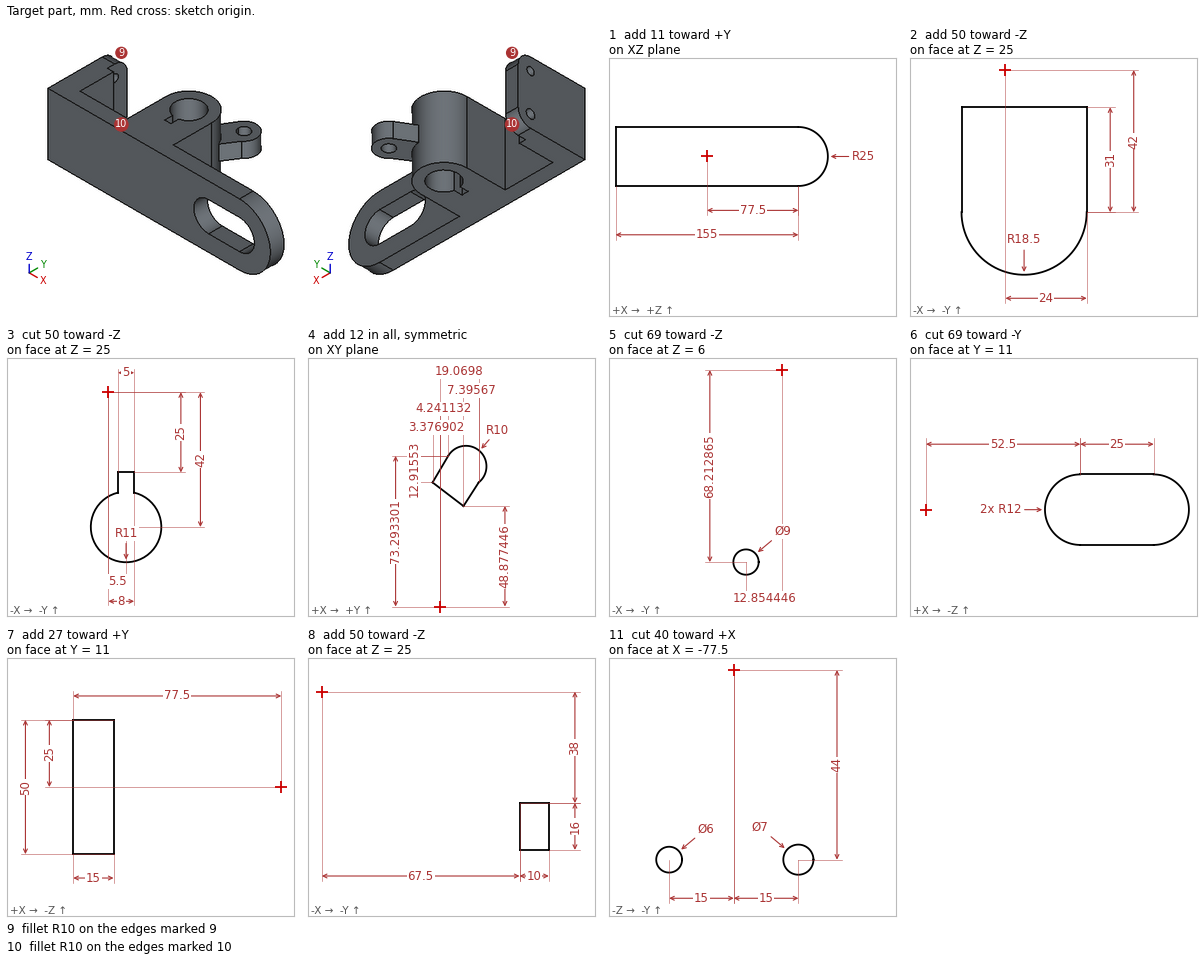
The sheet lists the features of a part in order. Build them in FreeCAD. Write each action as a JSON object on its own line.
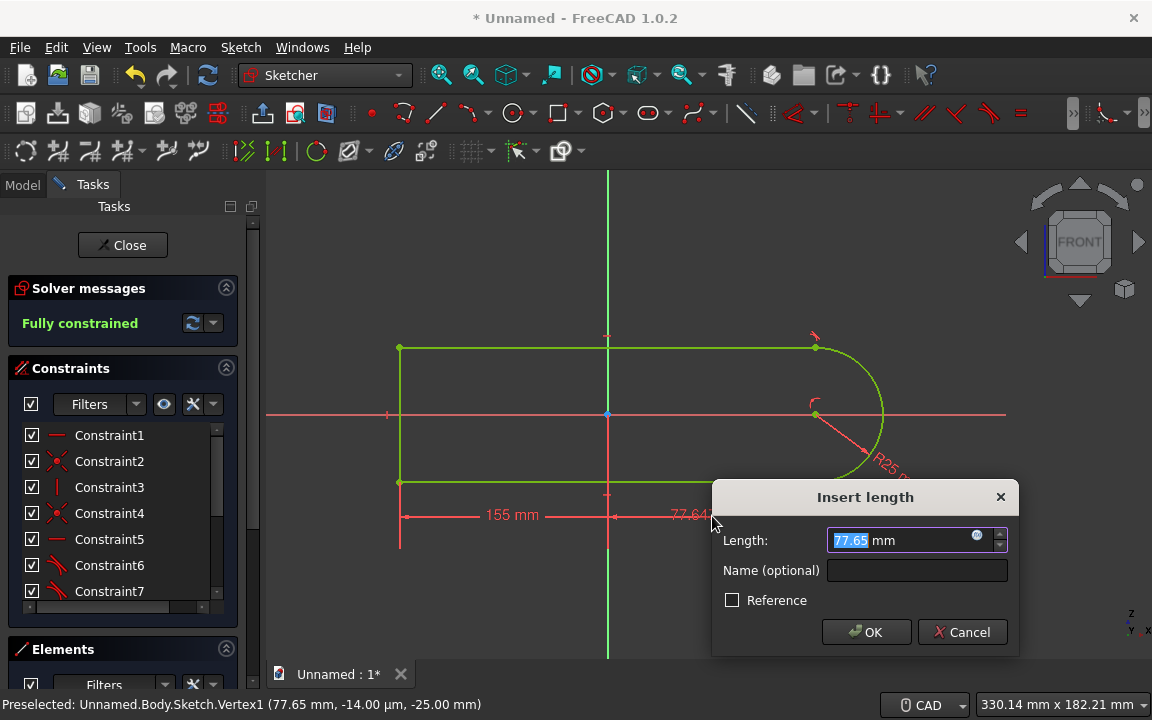
{"action": "type", "text": "77.5"}
{"action": "key", "text": "Return"}
{"action": "key", "text": "Escape"}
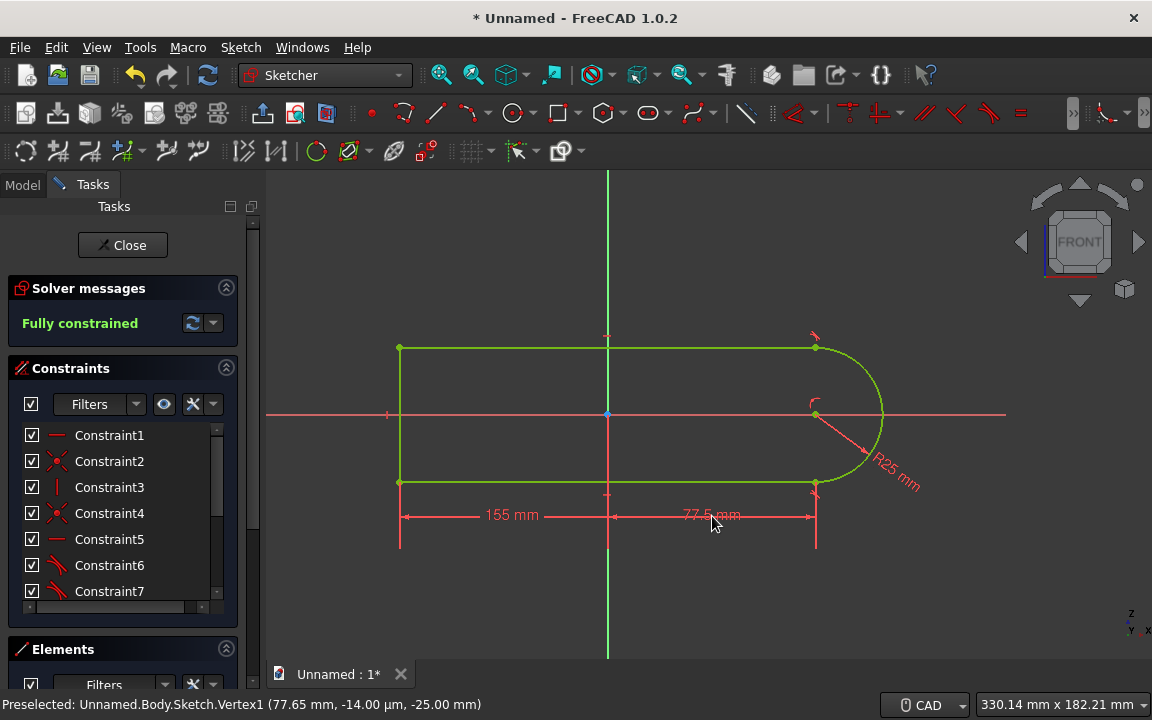
{"action": "left_click", "coordinate": [123, 245]}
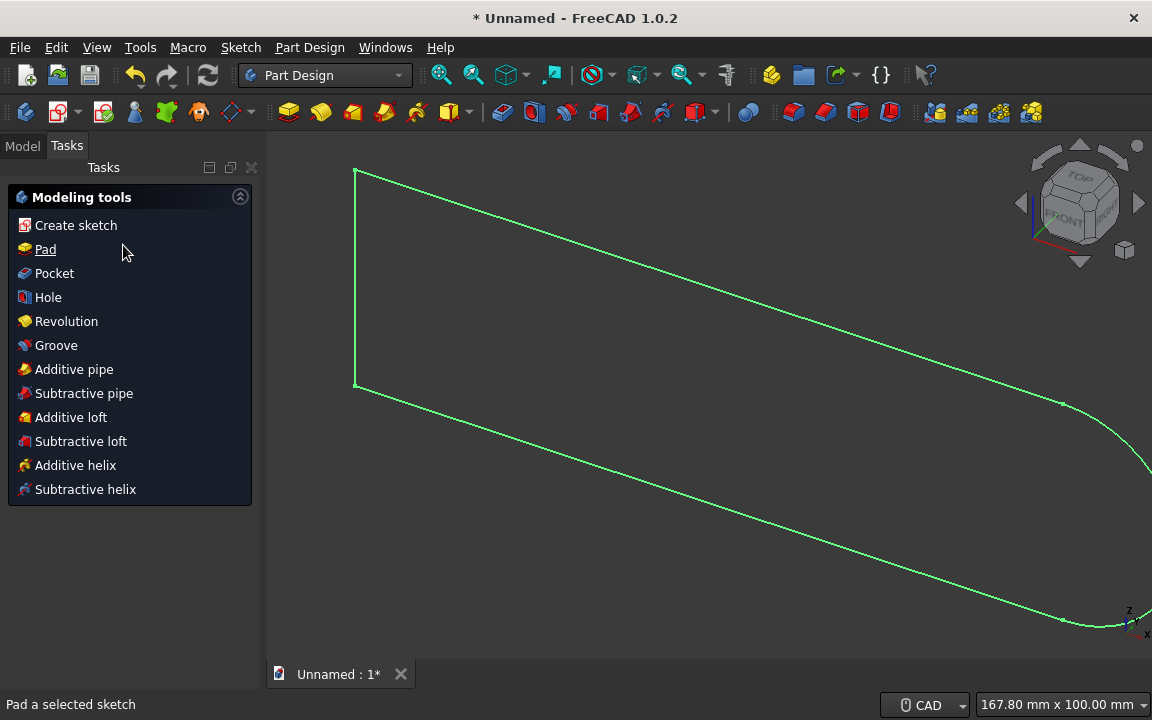
{"action": "left_click", "coordinate": [290, 112]}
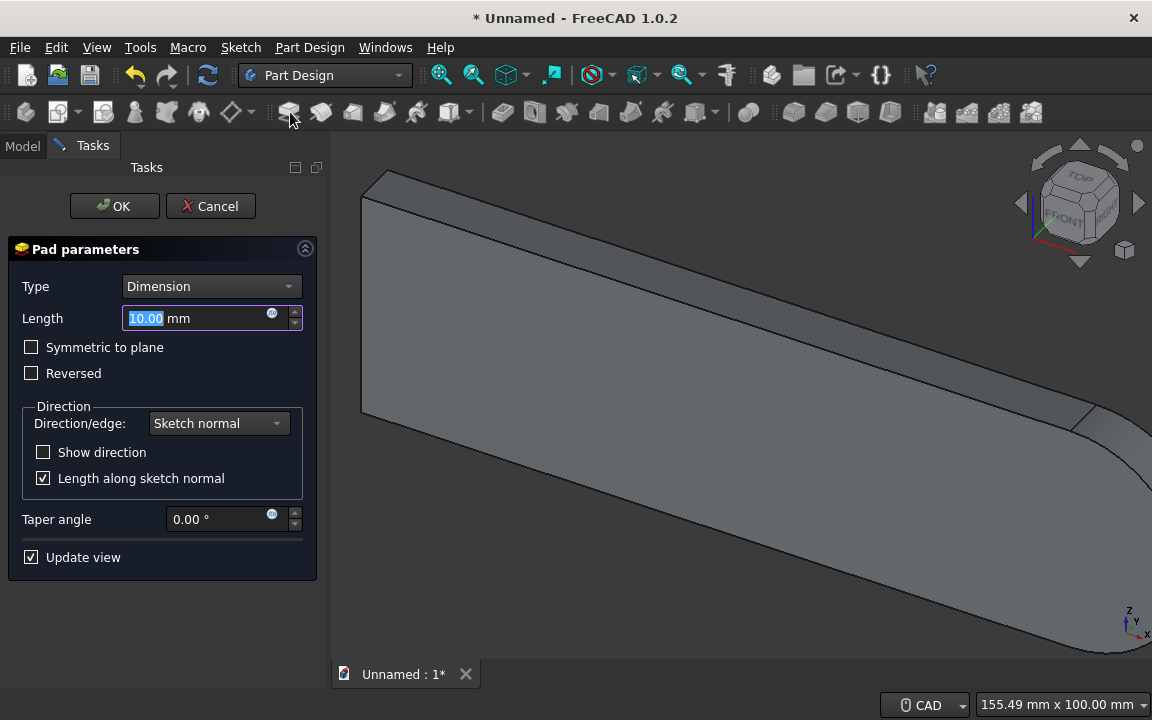
{"action": "type", "text": "11"}
{"action": "key", "text": "Tab"}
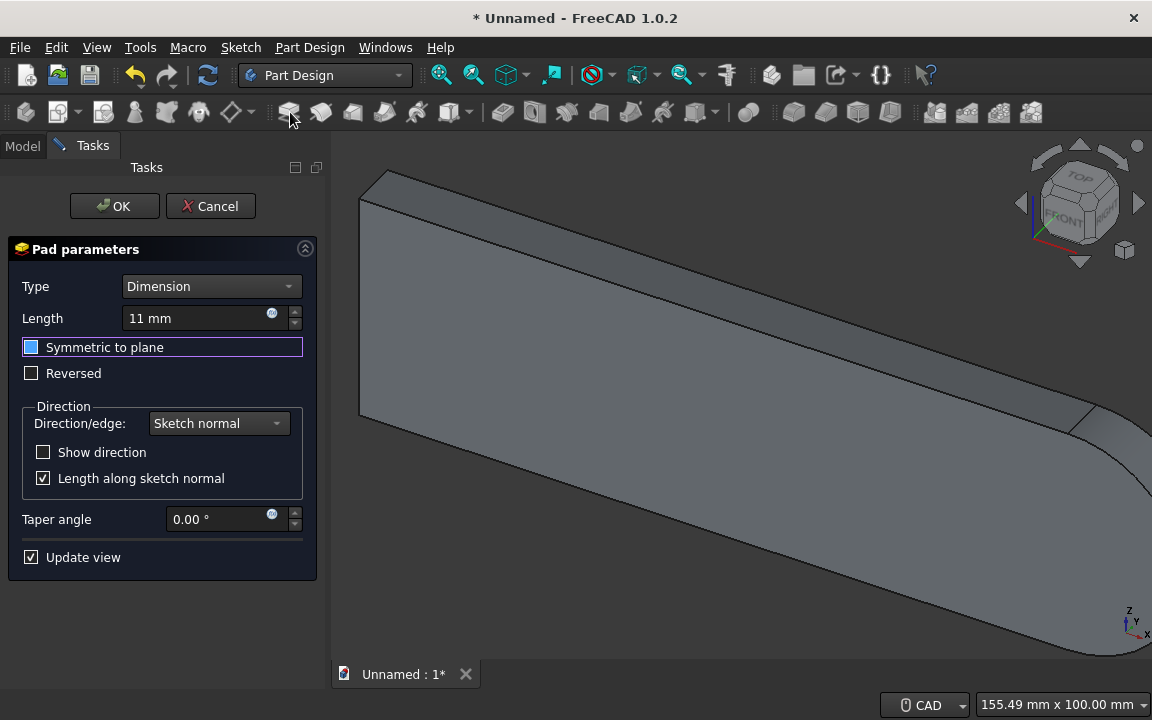
{"action": "left_click", "coordinate": [30, 373]}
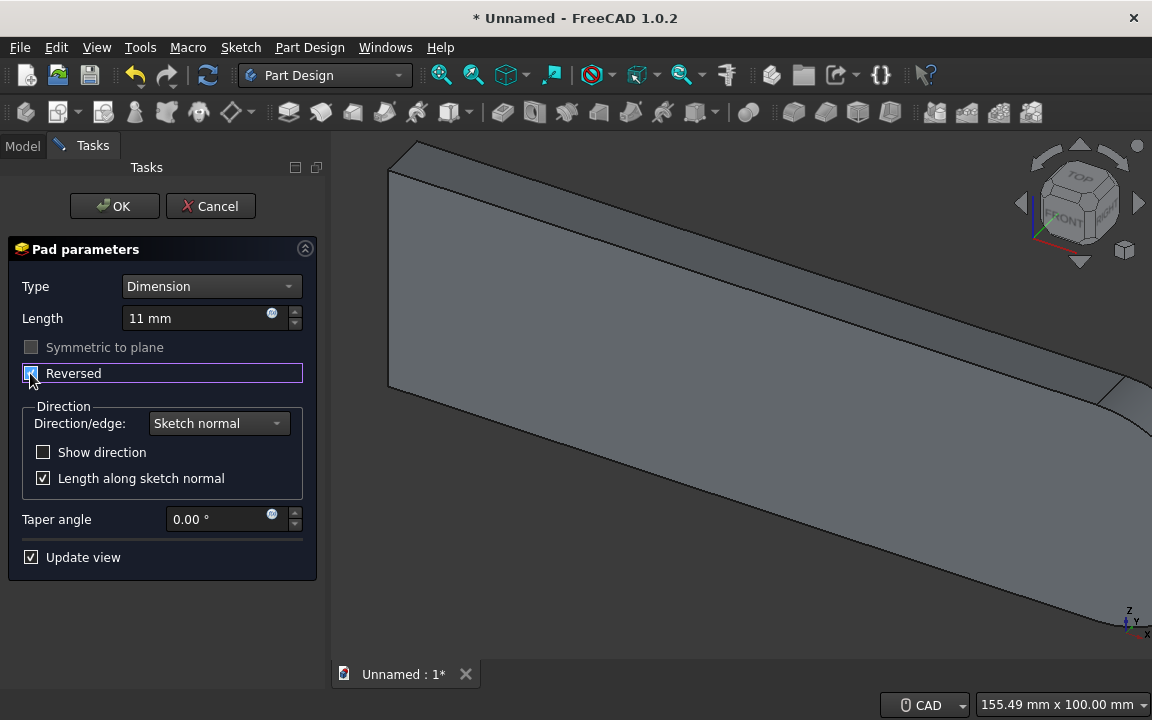
{"action": "left_click", "coordinate": [115, 206]}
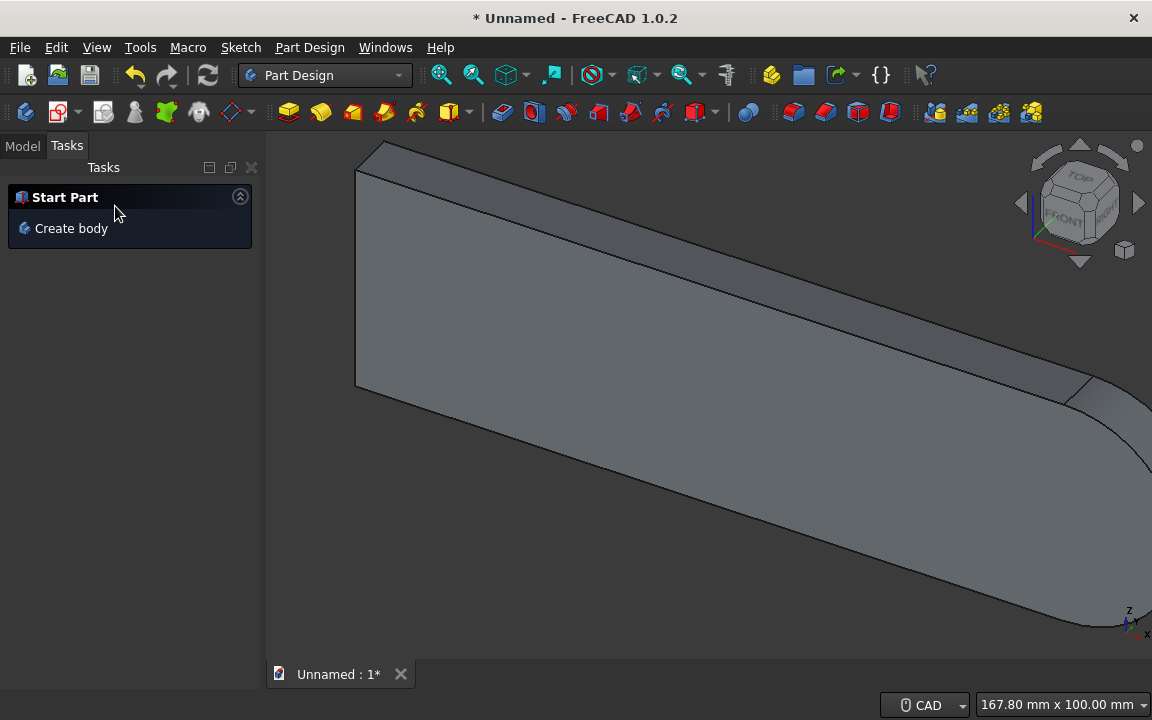
{"action": "left_click", "coordinate": [442, 76]}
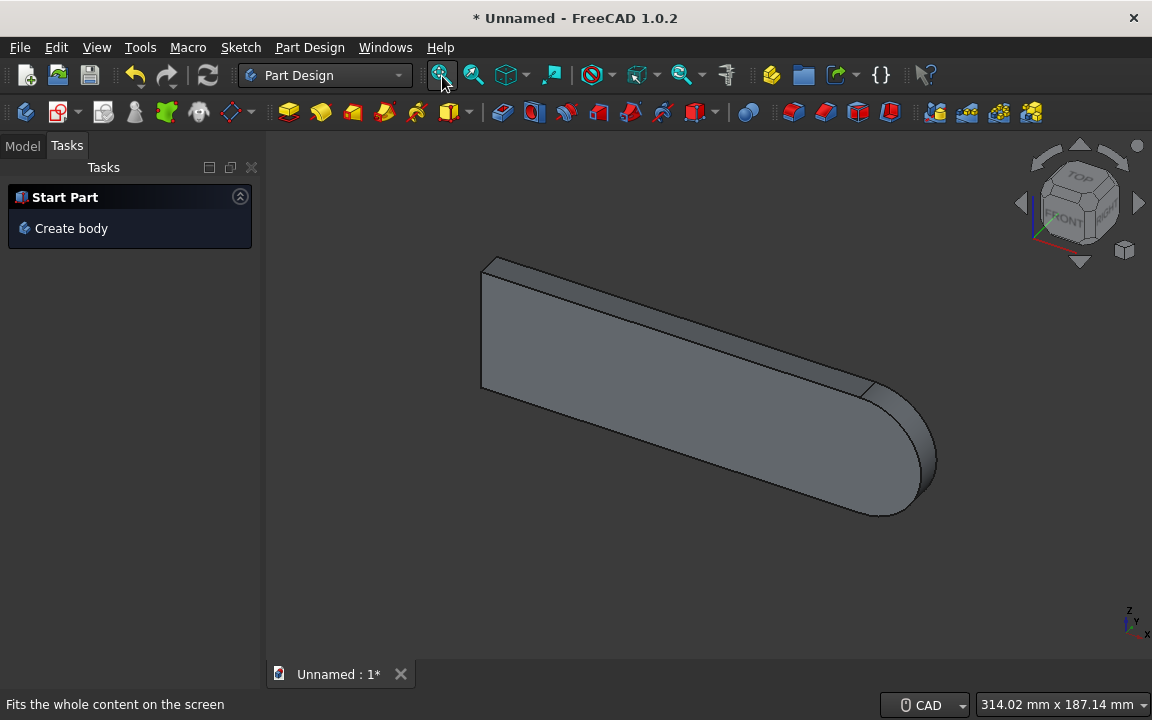
{"action": "left_click", "coordinate": [841, 380]}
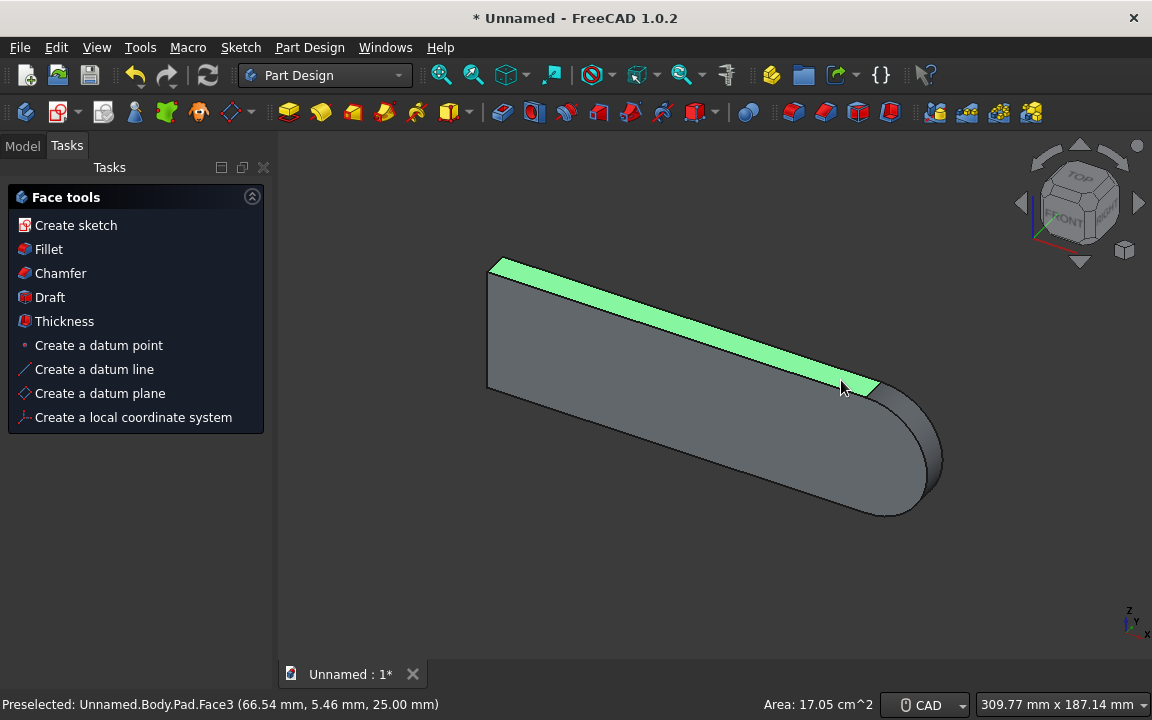
{"action": "left_click", "coordinate": [58, 112]}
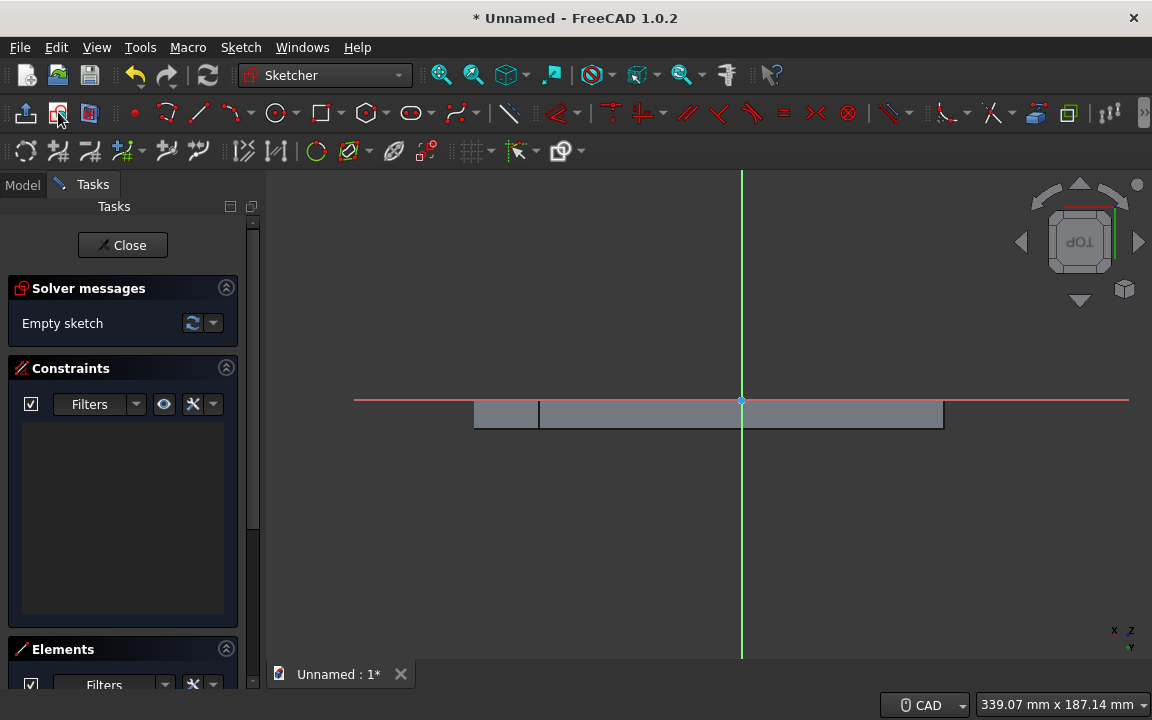
{"action": "scroll", "coordinate": [897, 558], "scroll_direction": "up", "scroll_amount": 3}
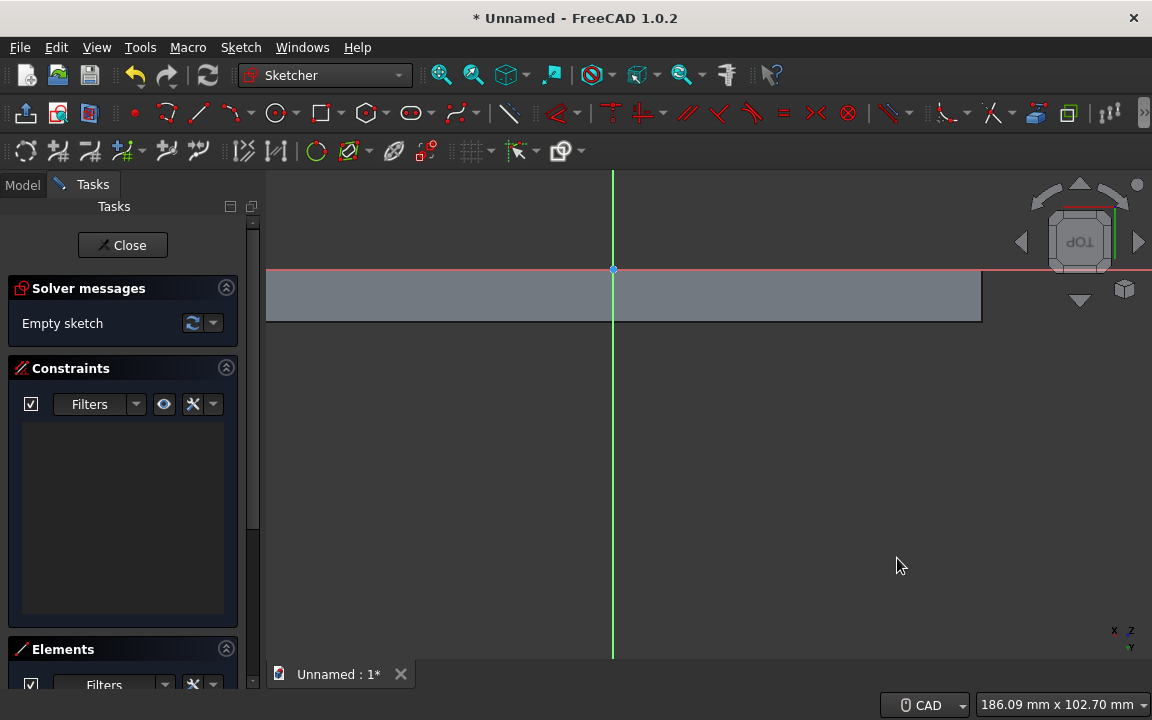
{"action": "left_click", "coordinate": [168, 114]}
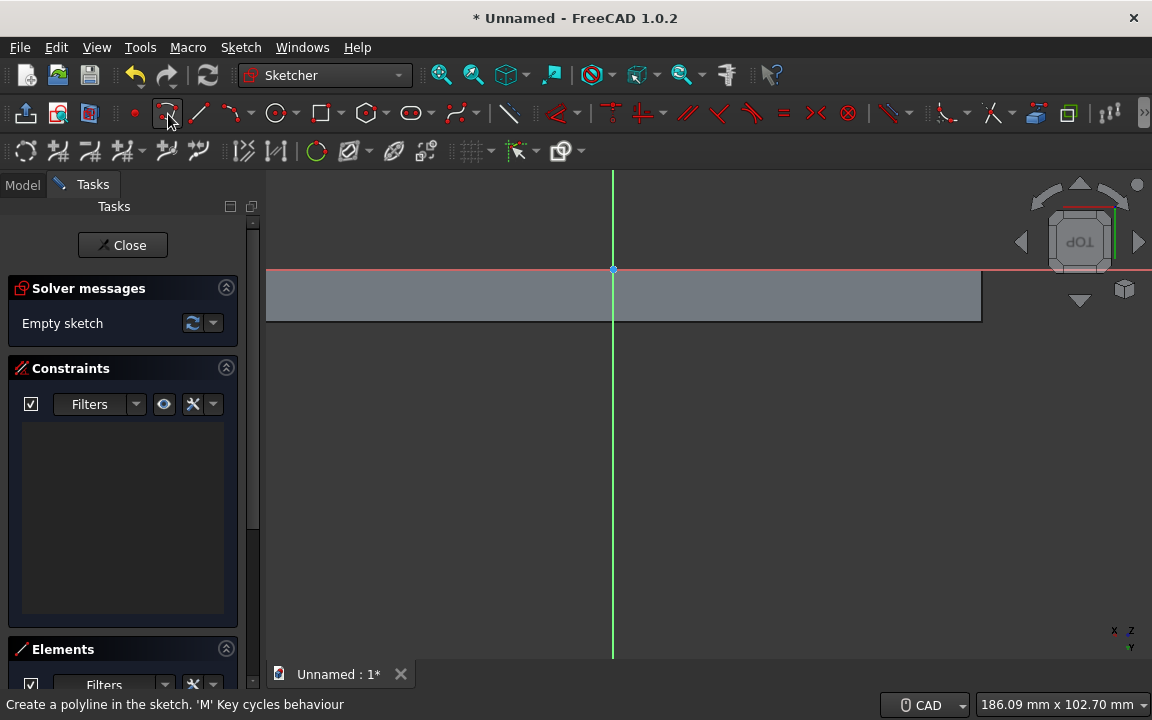
{"action": "left_click", "coordinate": [728, 470]}
{"action": "left_click", "coordinate": [728, 322]}
{"action": "left_click", "coordinate": [551, 322]}
{"action": "left_click", "coordinate": [551, 470]}
{"action": "right_click", "coordinate": [551, 470]}